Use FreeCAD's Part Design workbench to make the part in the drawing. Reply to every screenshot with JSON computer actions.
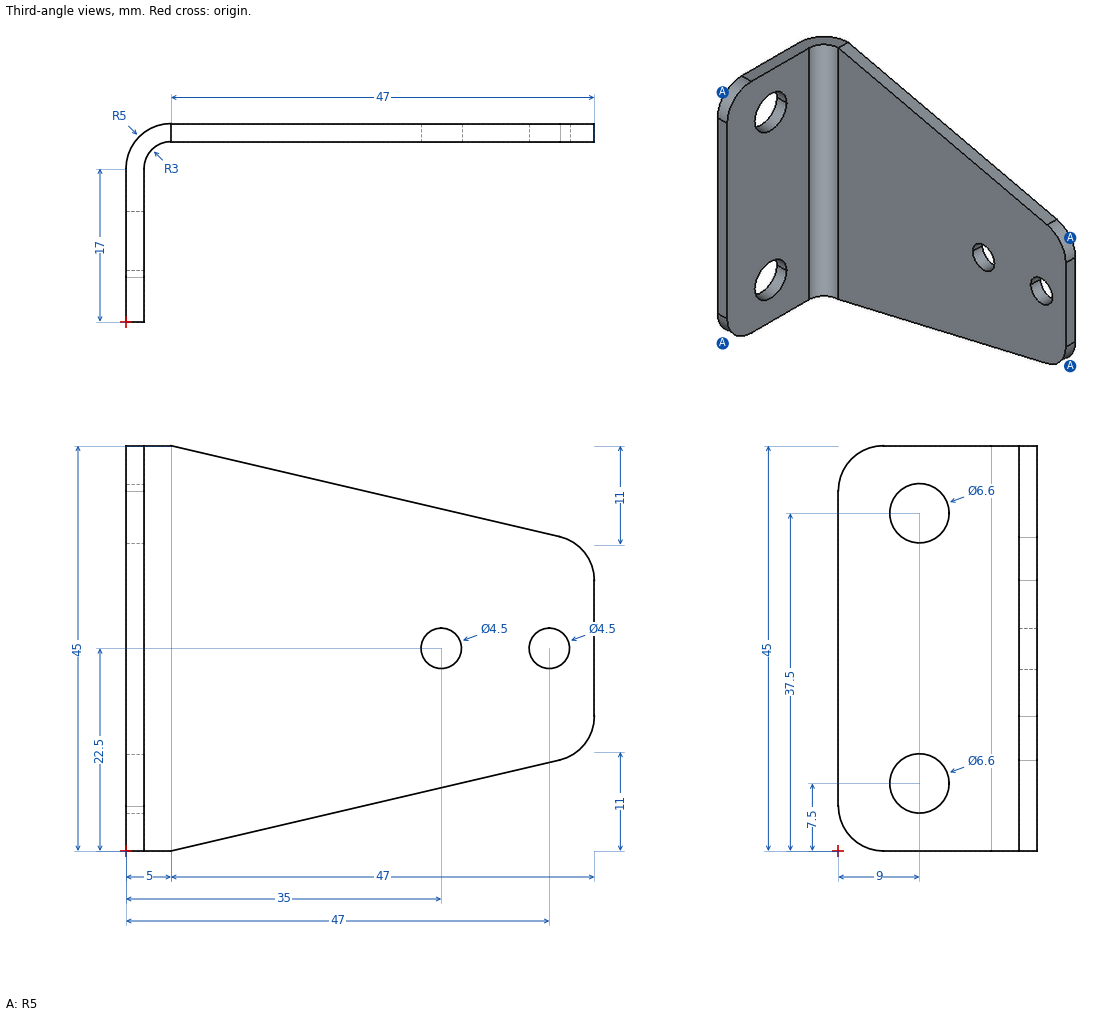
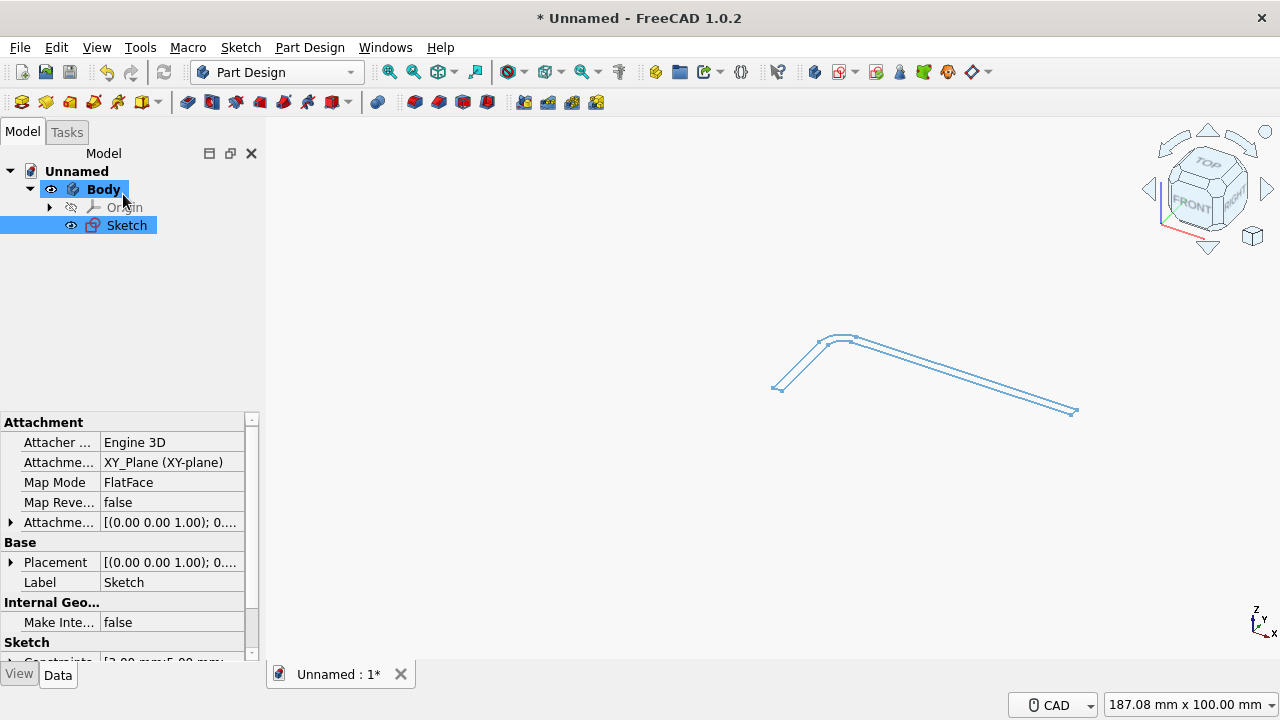
{"action": "left_click", "coordinate": [22, 102]}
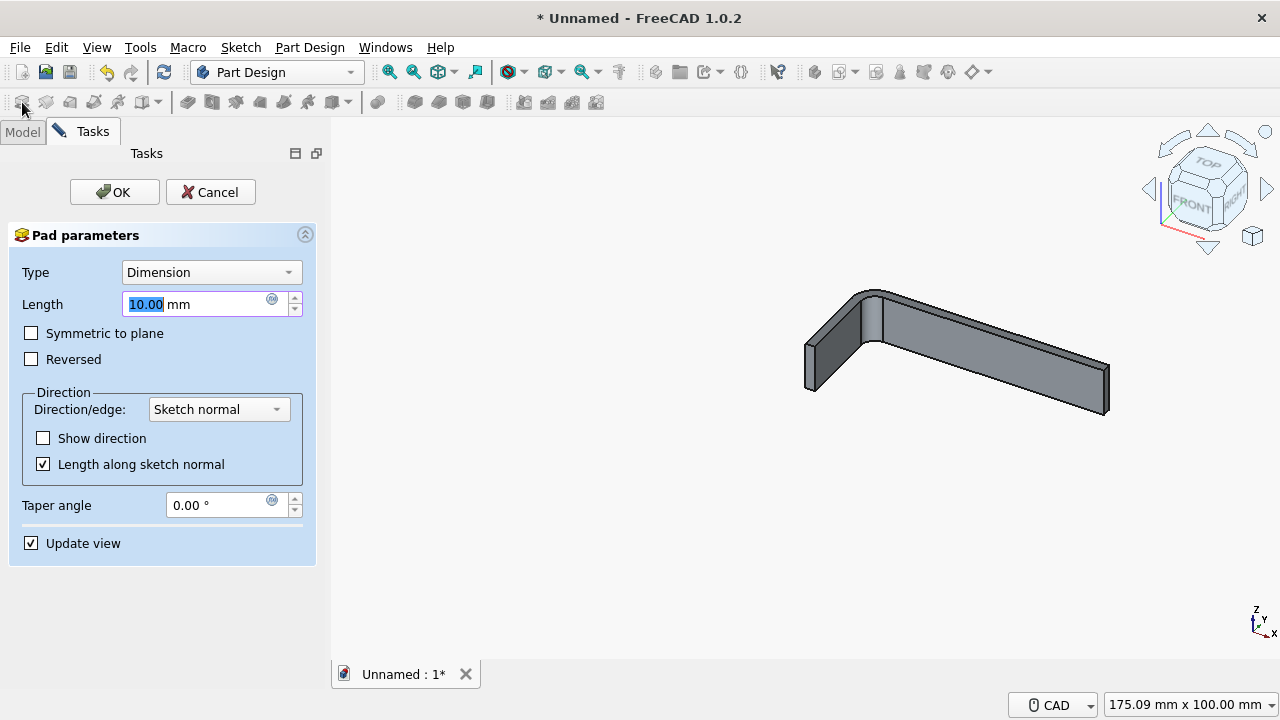
{"action": "type", "text": "45"}
{"action": "key", "text": "Tab"}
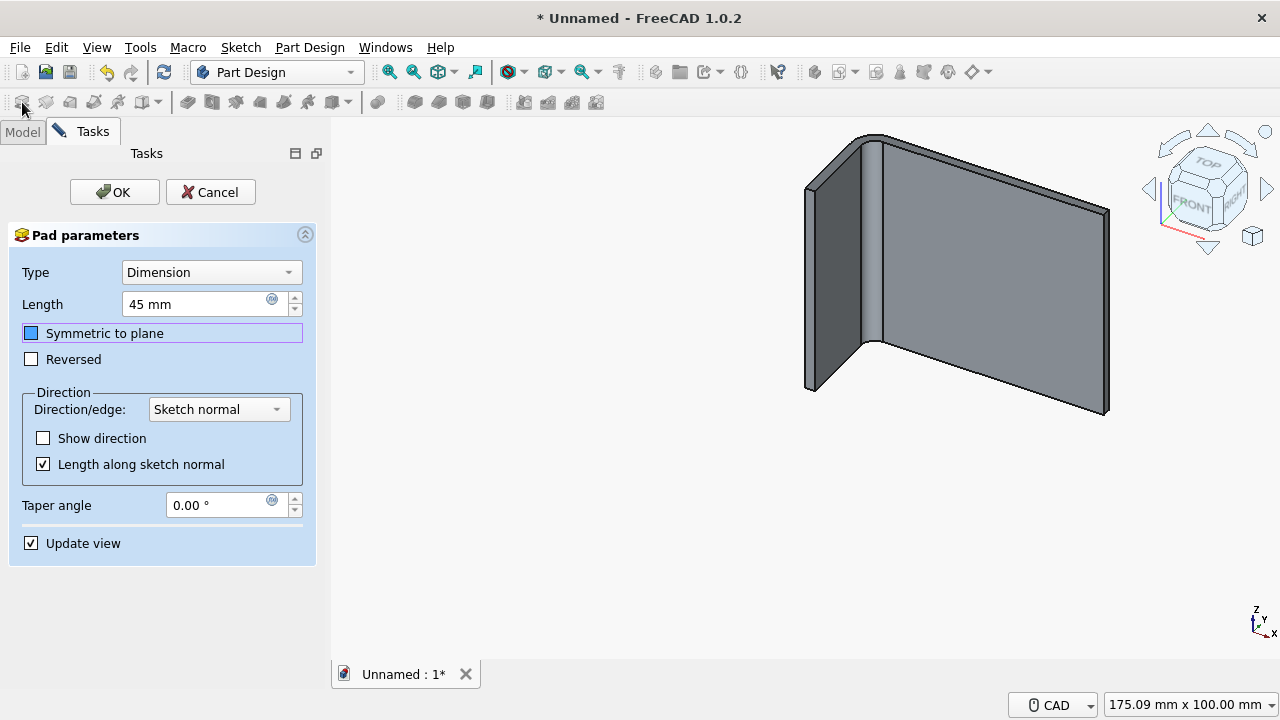
{"action": "left_click", "coordinate": [115, 192]}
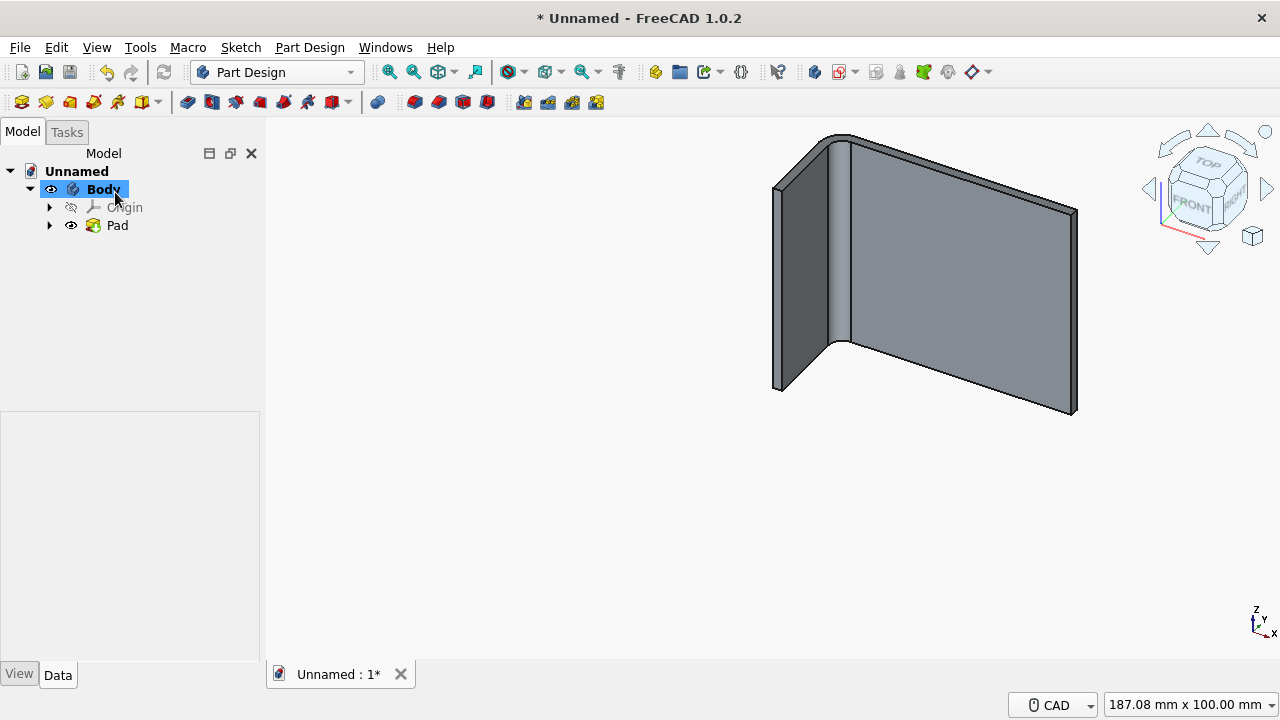
{"action": "left_click", "coordinate": [805, 210]}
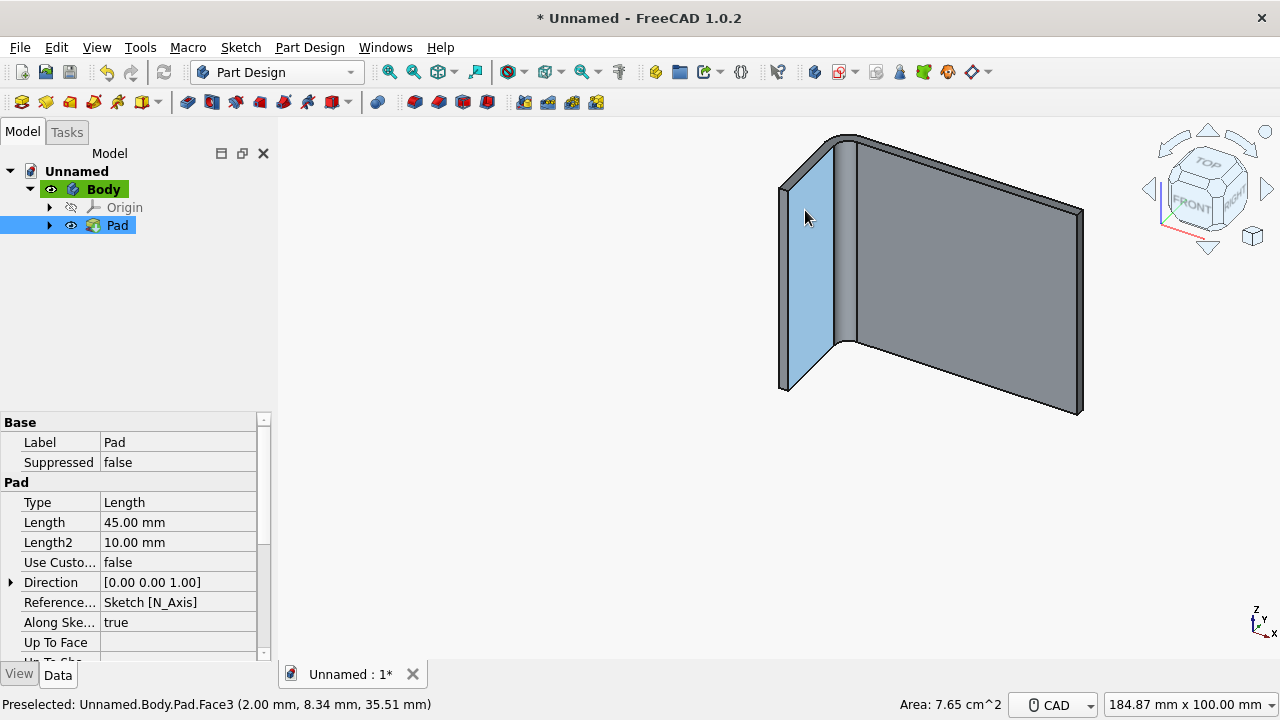
{"action": "left_click", "coordinate": [840, 72]}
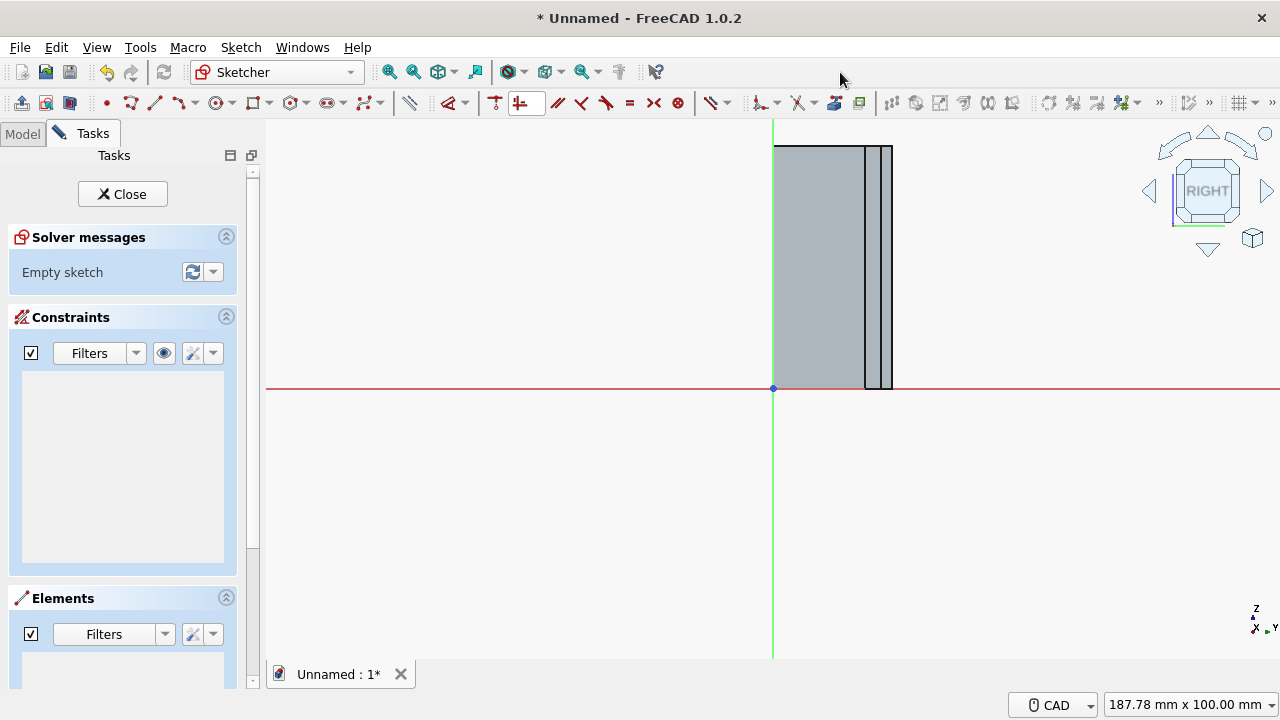
{"action": "key", "text": "q s"}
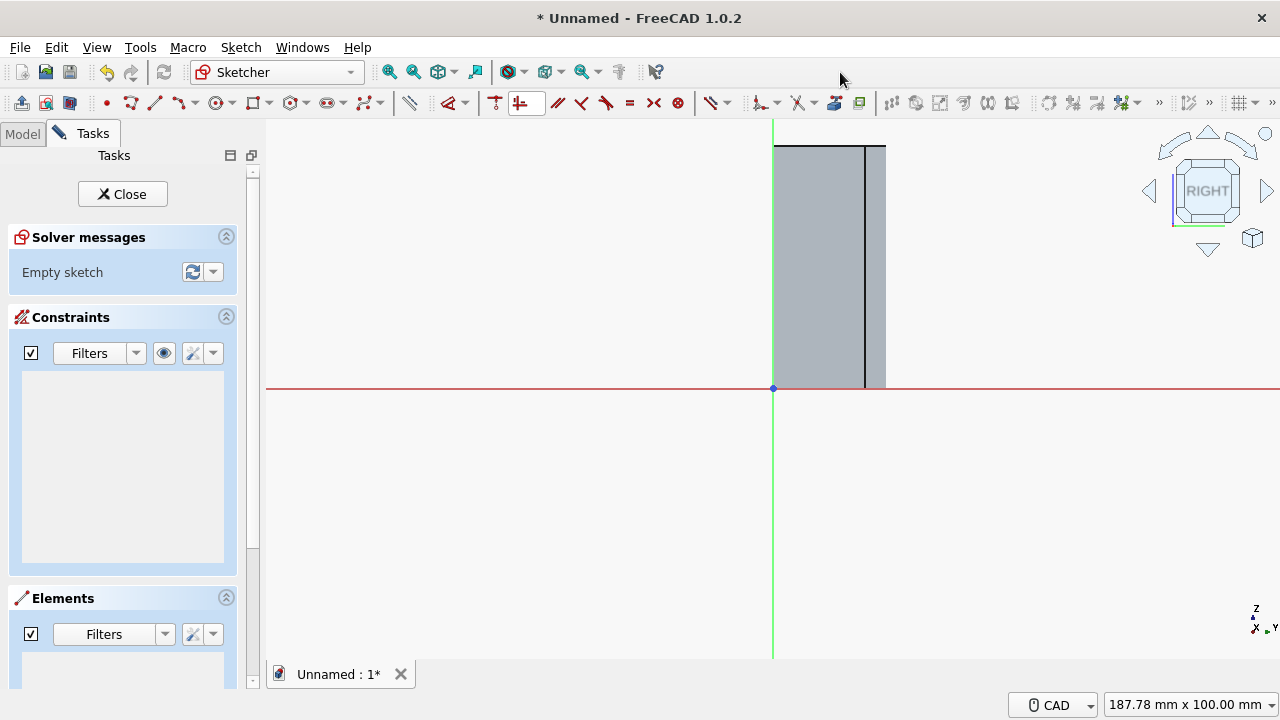
{"action": "scroll", "coordinate": [836, 161], "scroll_direction": "up", "scroll_amount": 11}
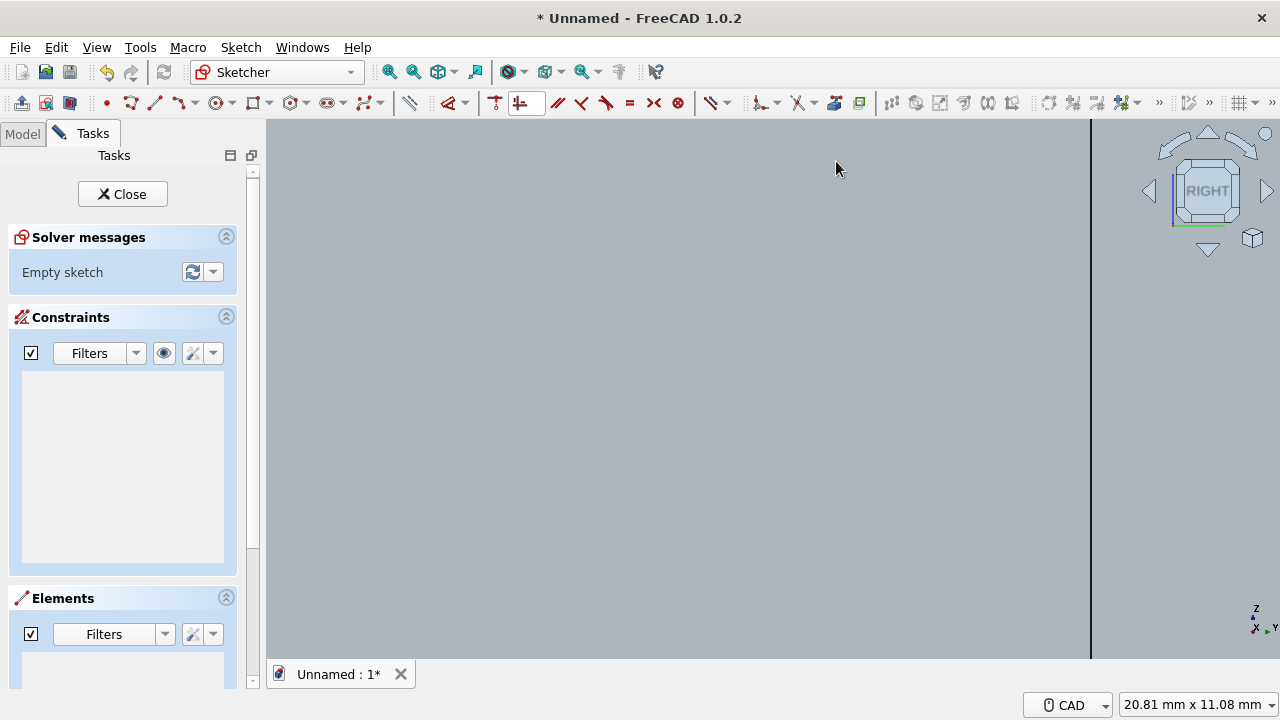
{"action": "left_click", "coordinate": [216, 104]}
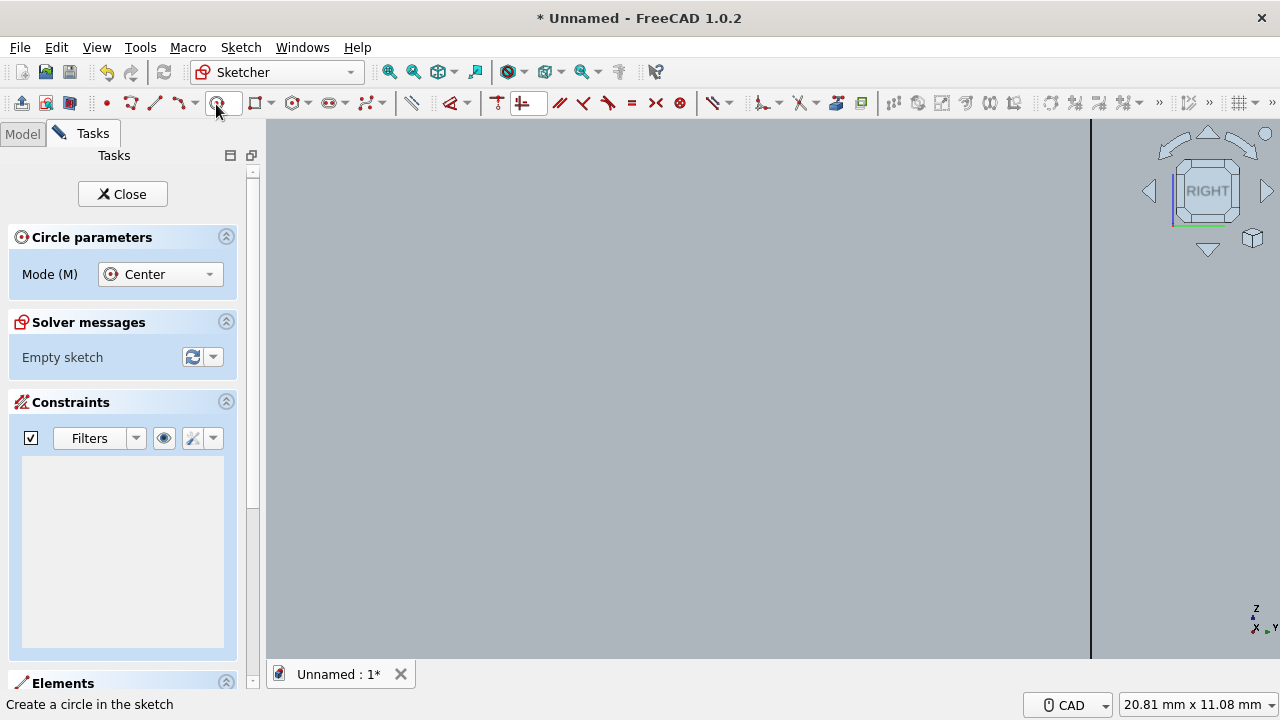
{"action": "left_click", "coordinate": [702, 391]}
{"action": "mouse_move", "coordinate": [815, 277]}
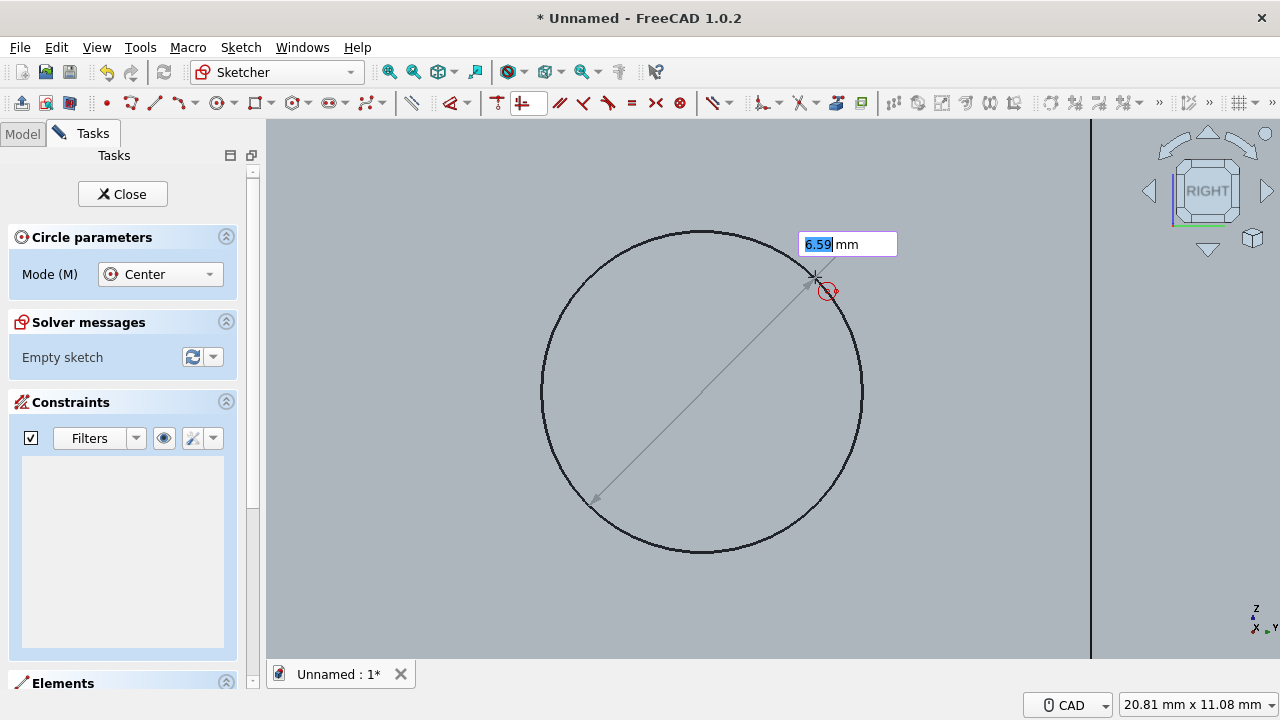
{"action": "type", "text": "6.6"}
{"action": "key", "text": "Return"}
{"action": "key", "text": "Escape"}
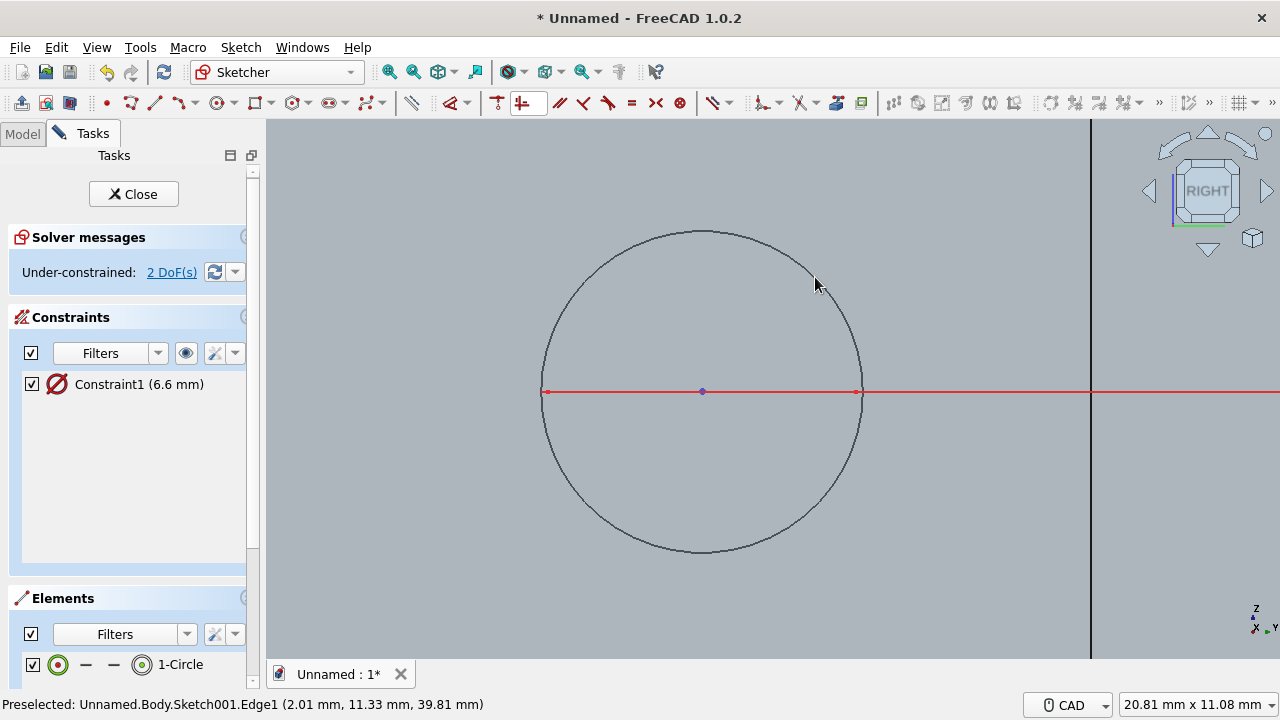
{"action": "key", "text": "d"}